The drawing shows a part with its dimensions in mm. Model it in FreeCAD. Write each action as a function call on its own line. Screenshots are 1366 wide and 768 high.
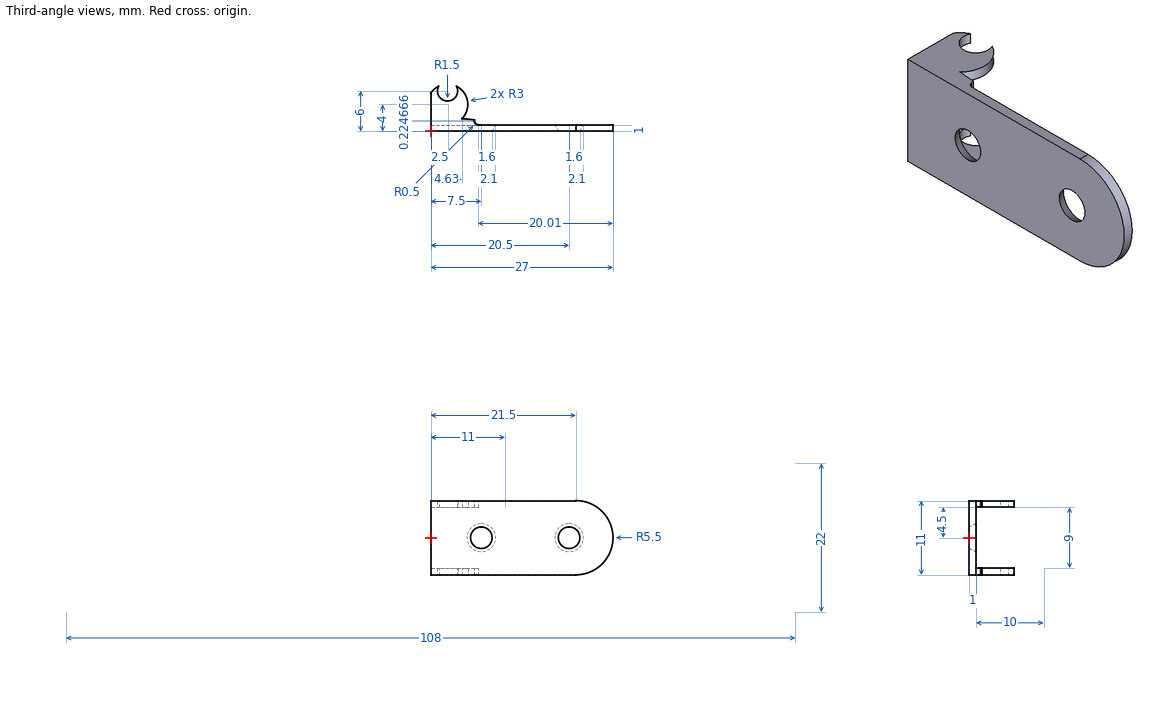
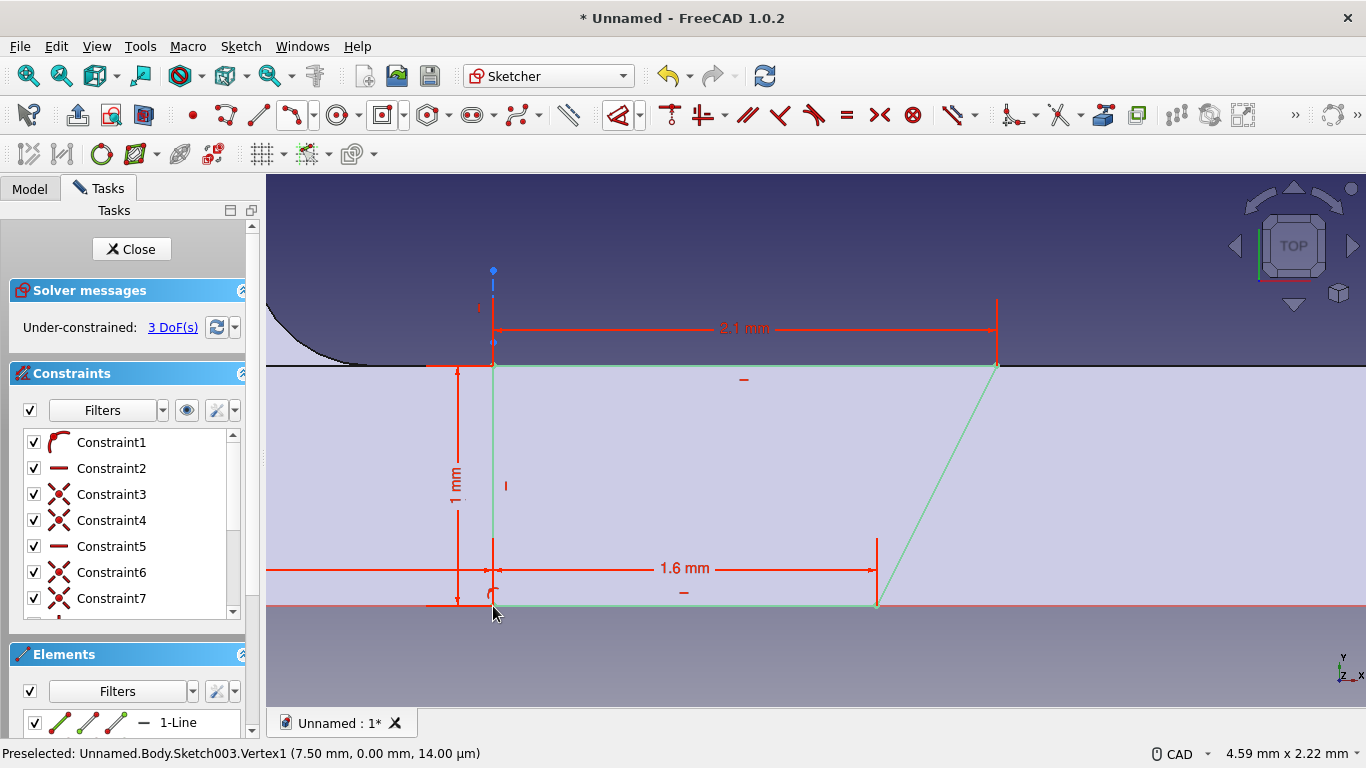
click(493, 343)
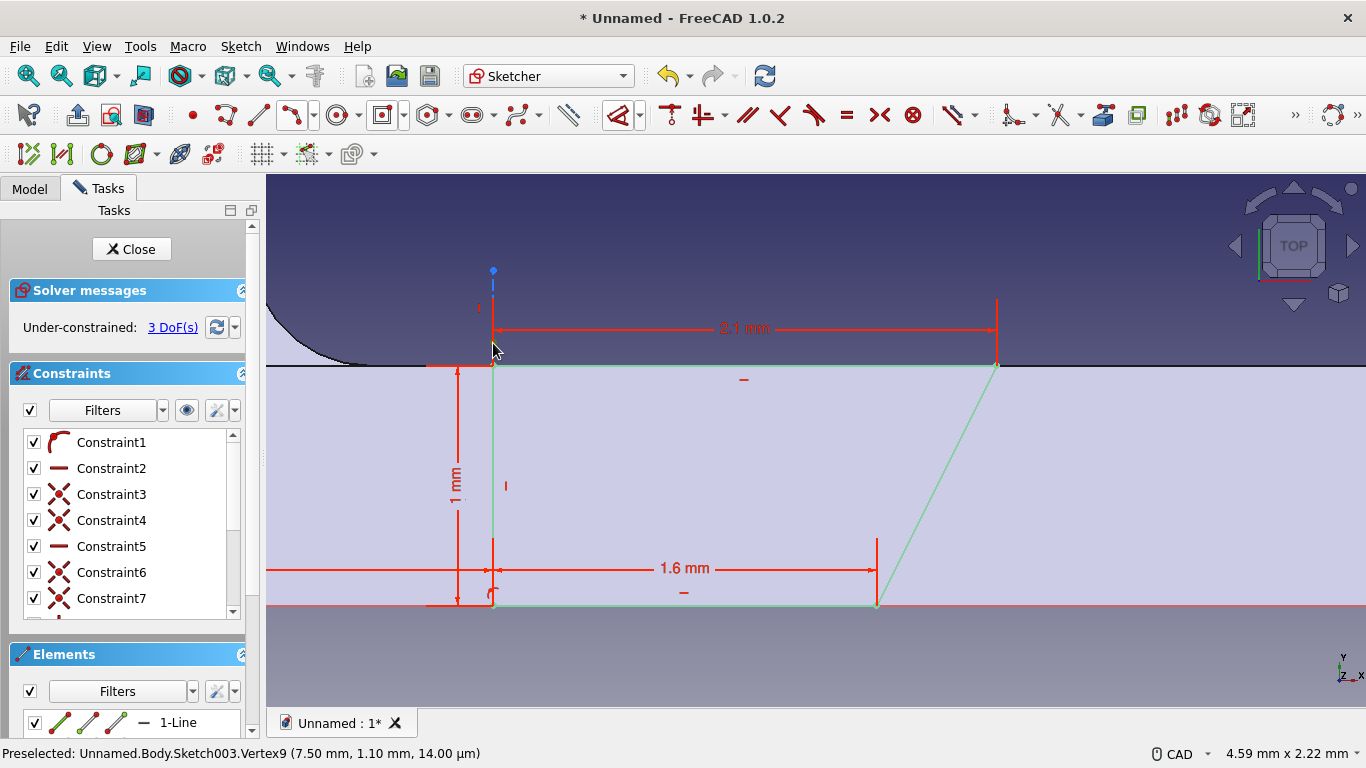
click(640, 116)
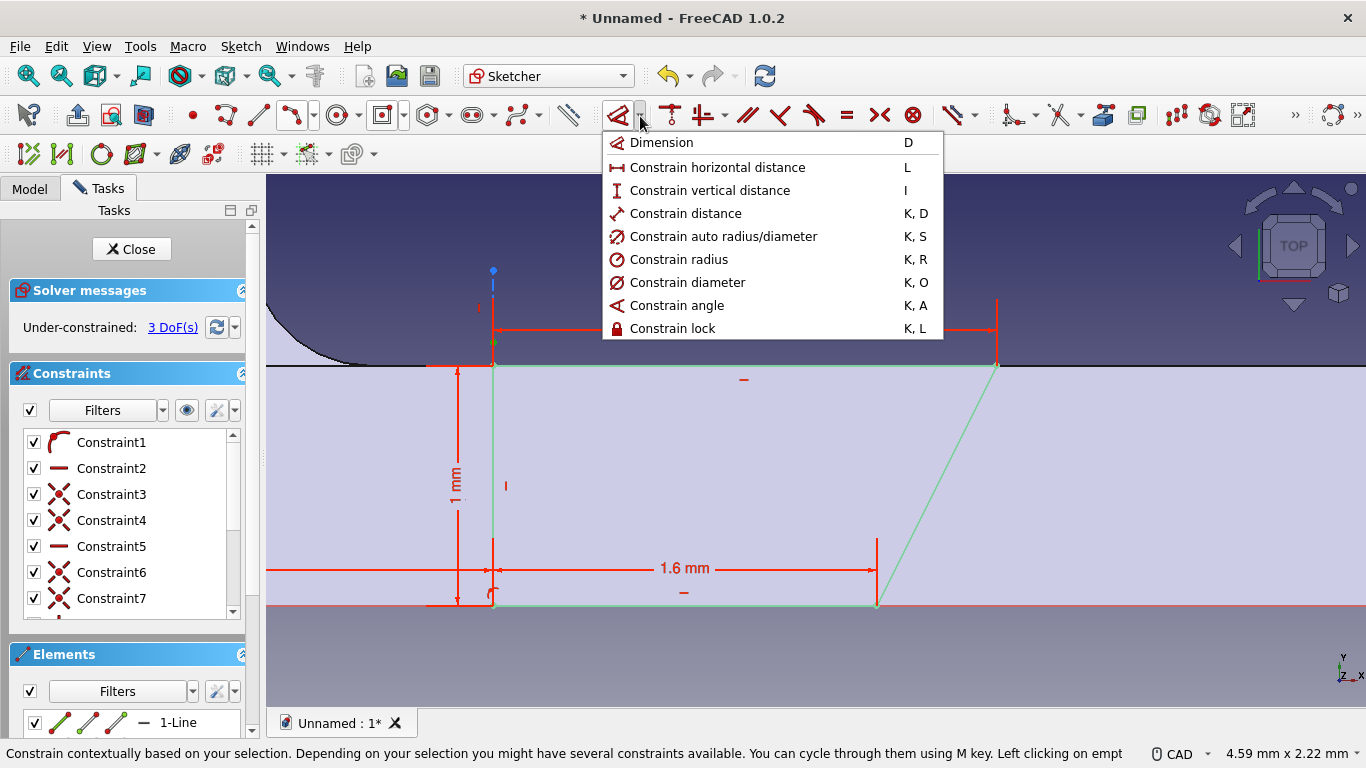
click(773, 168)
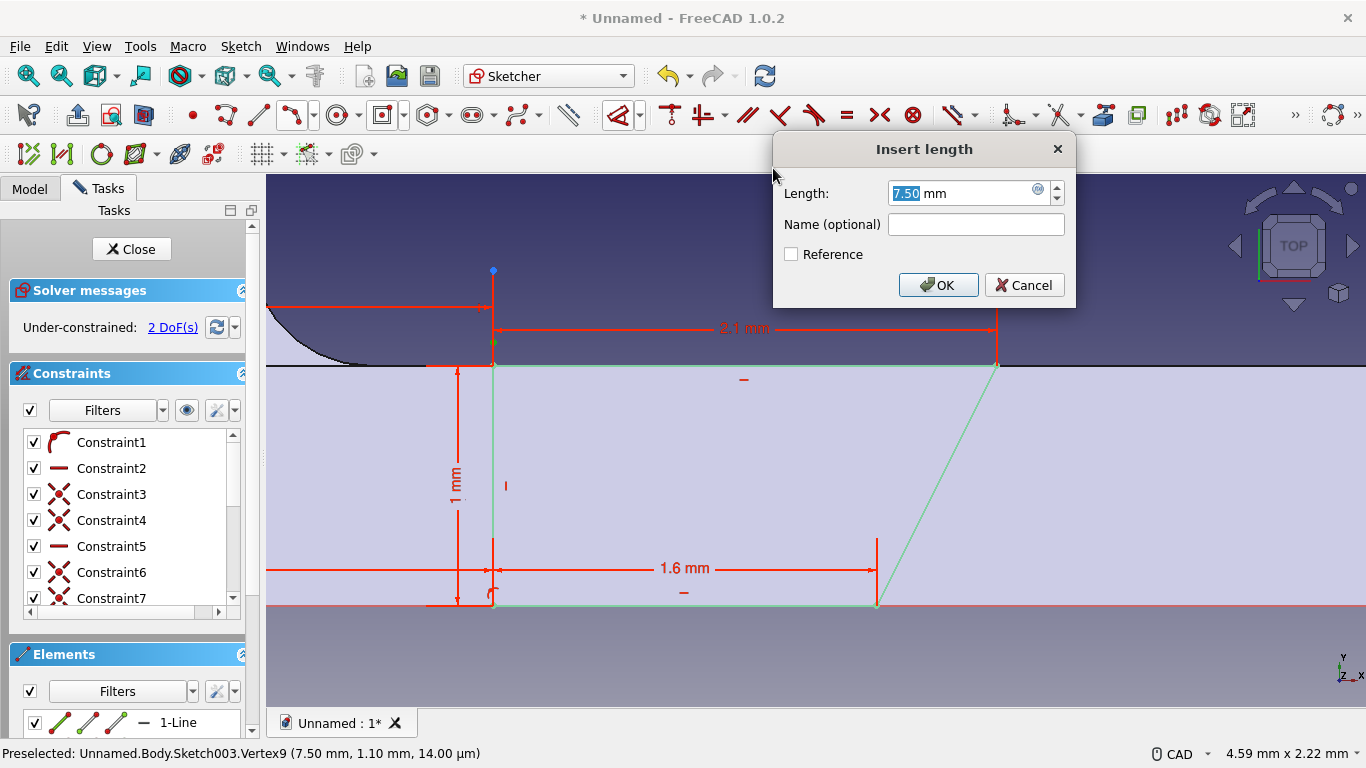
text(7.5)
key(Return)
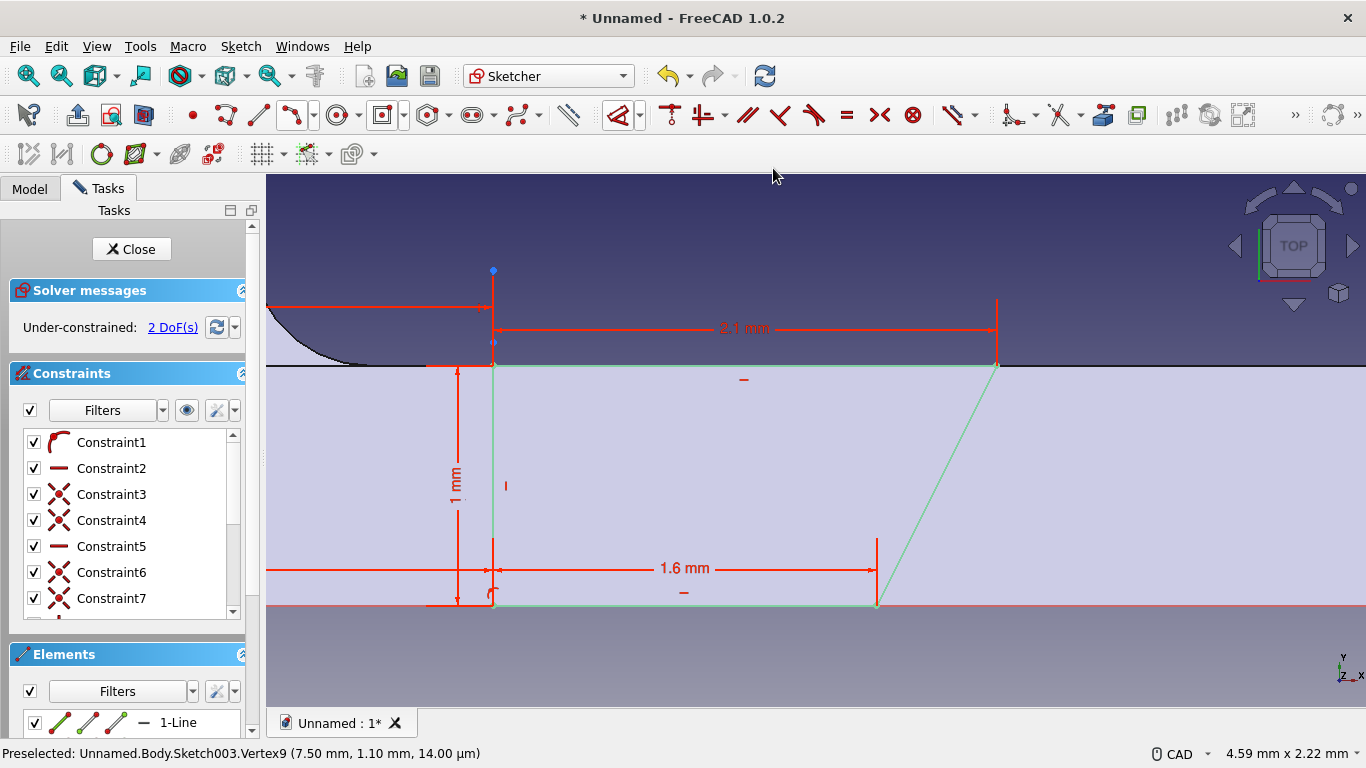
click(132, 249)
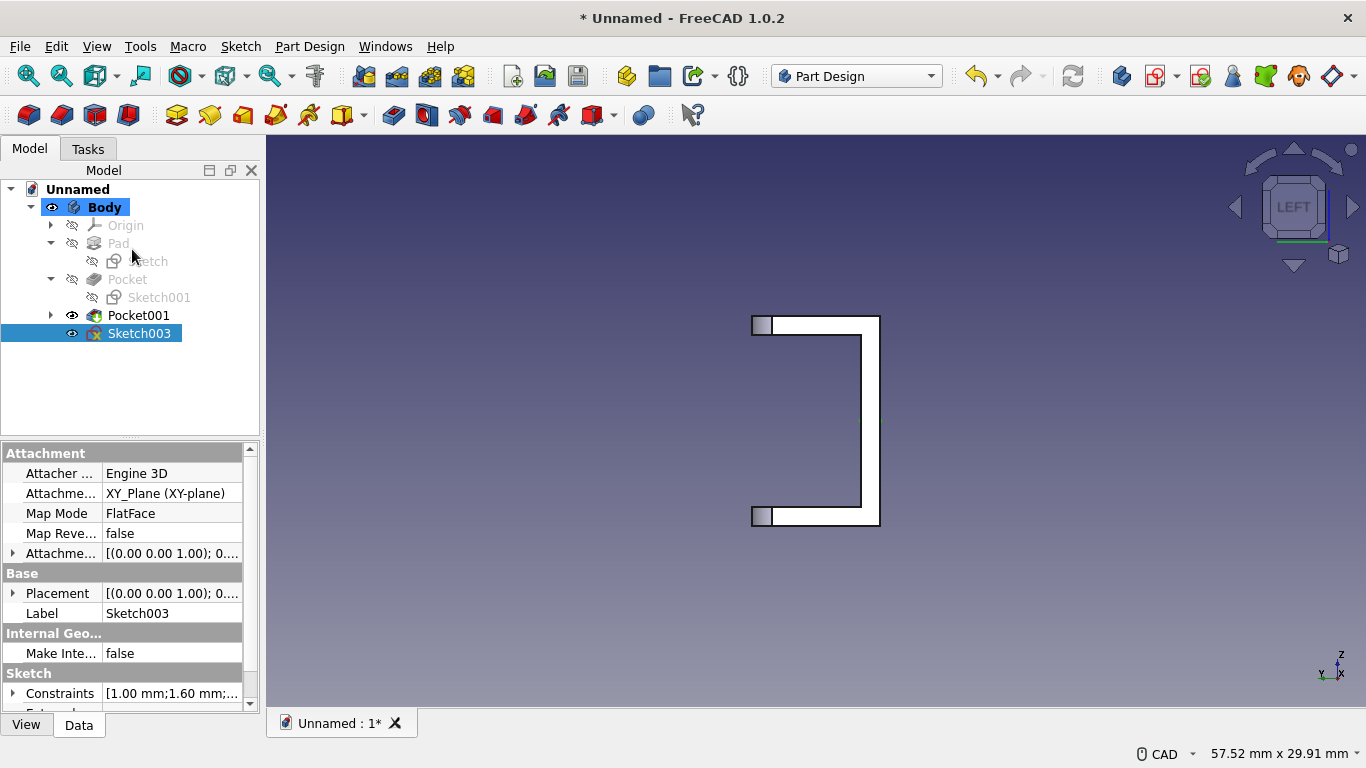
click(460, 116)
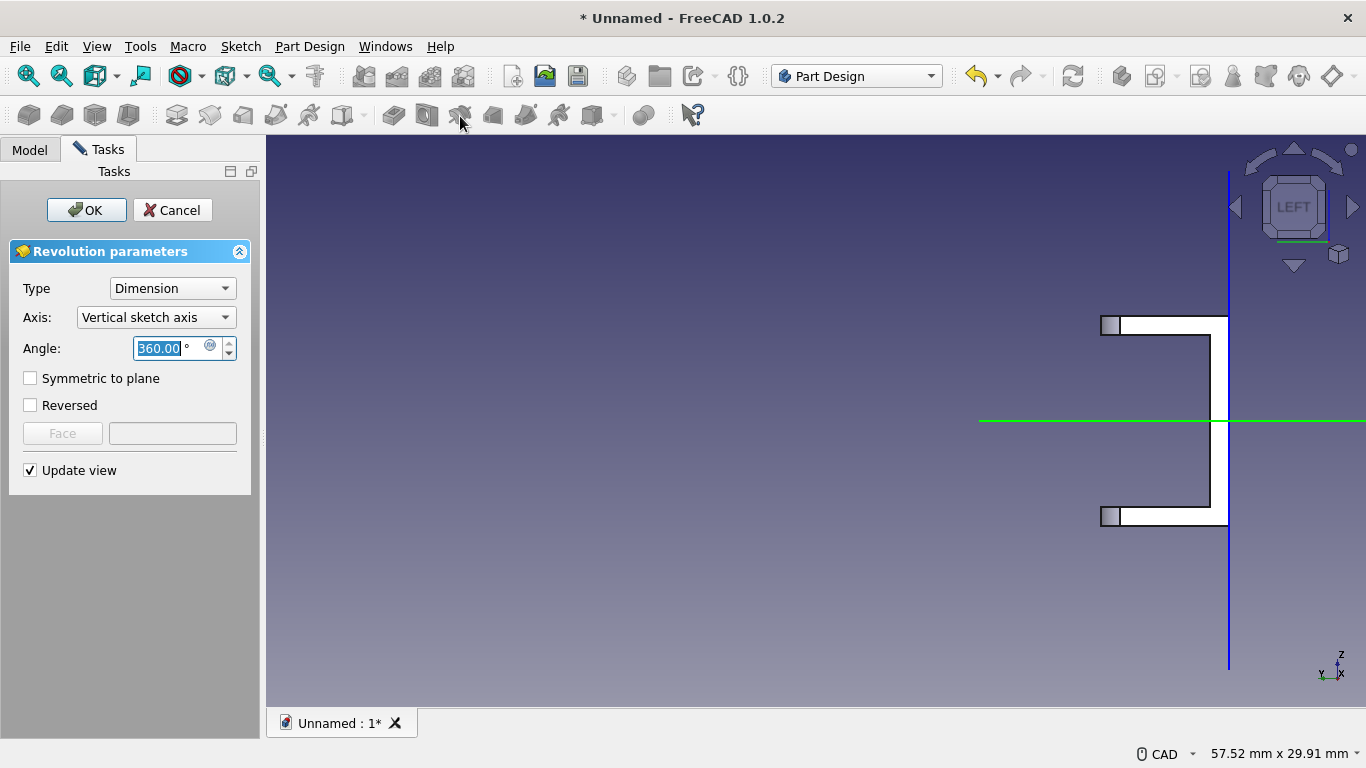
click(157, 318)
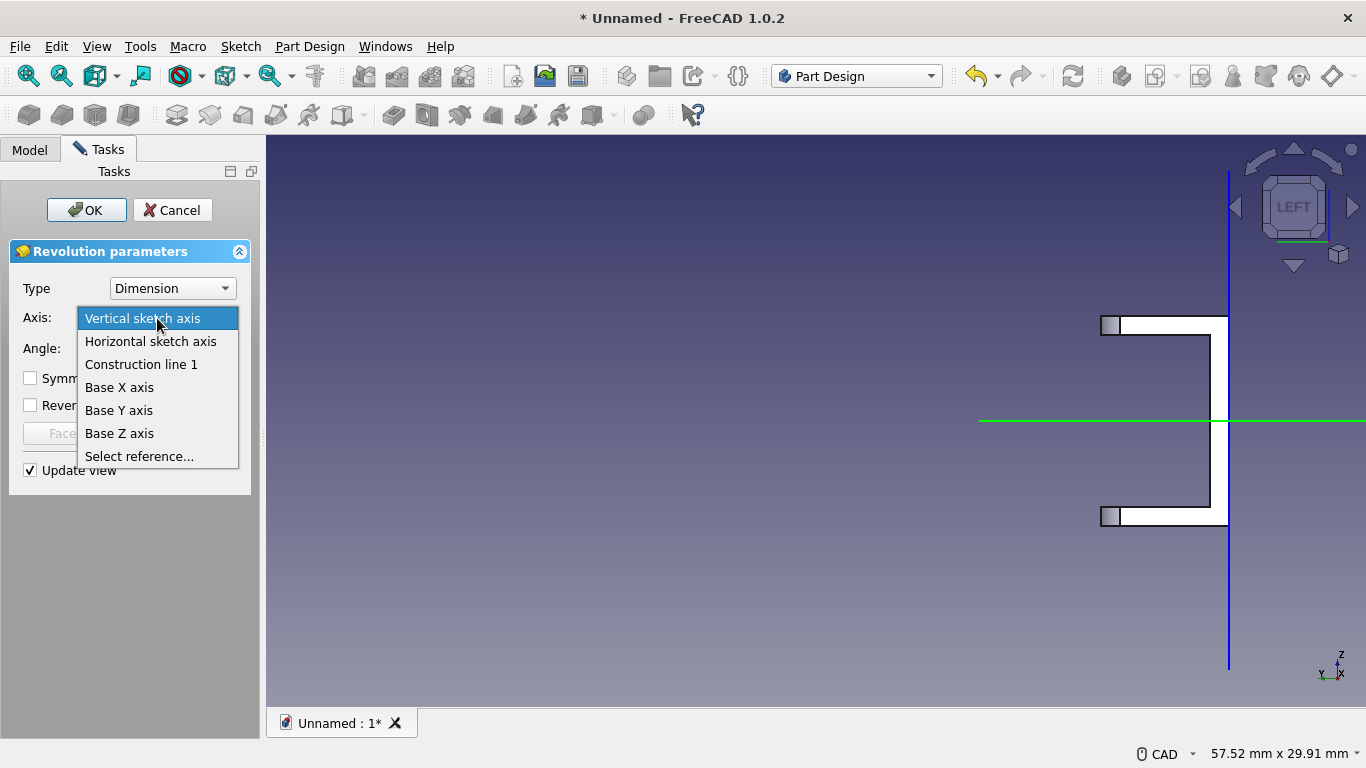
click(156, 364)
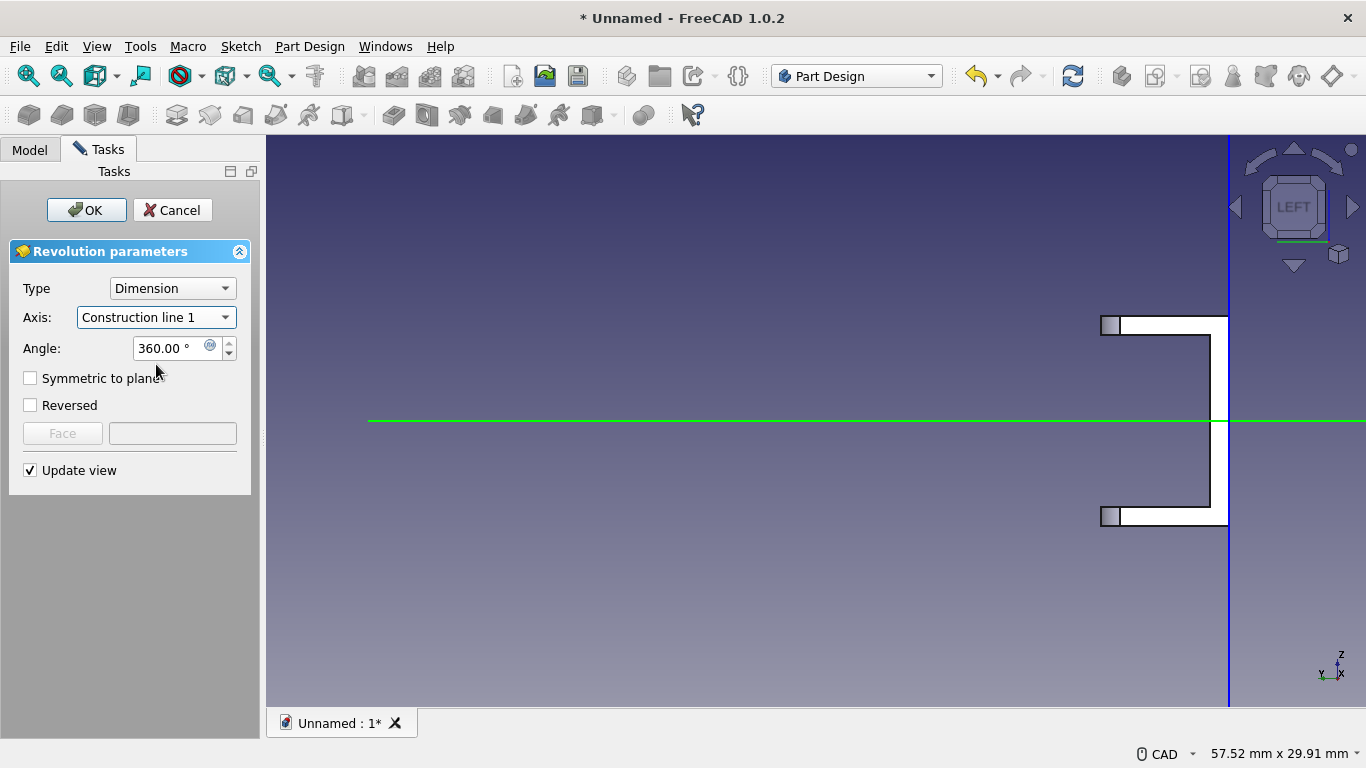
click(87, 210)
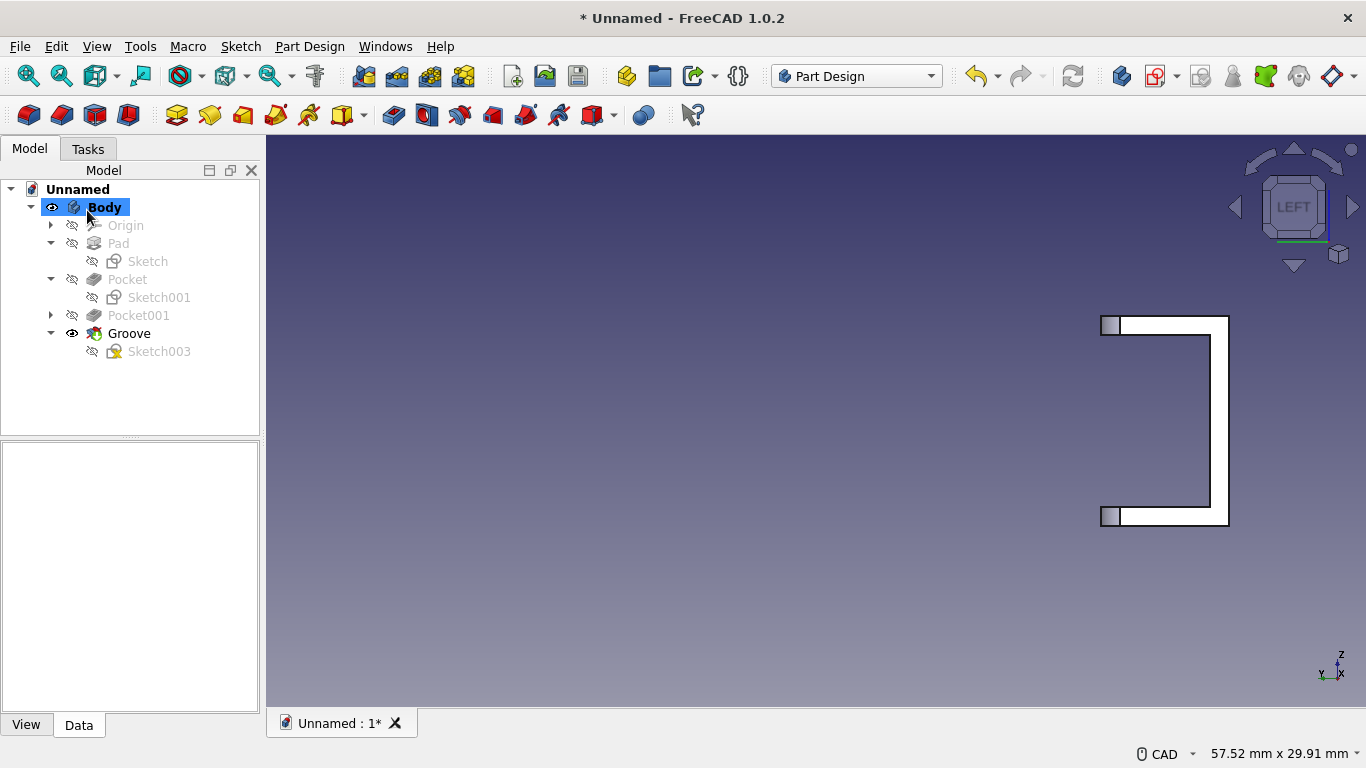
click(29, 76)